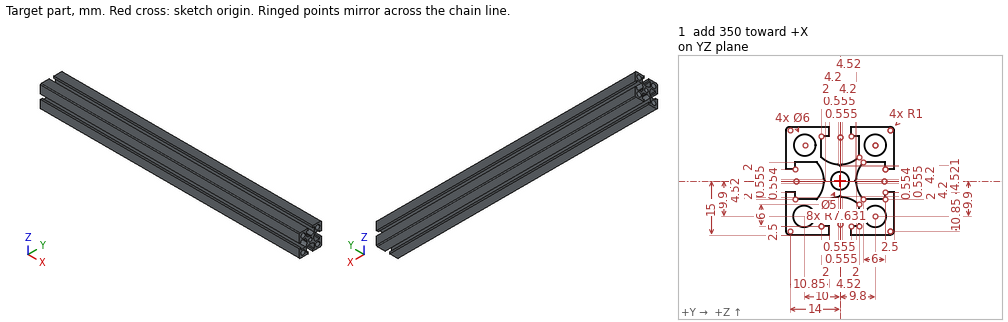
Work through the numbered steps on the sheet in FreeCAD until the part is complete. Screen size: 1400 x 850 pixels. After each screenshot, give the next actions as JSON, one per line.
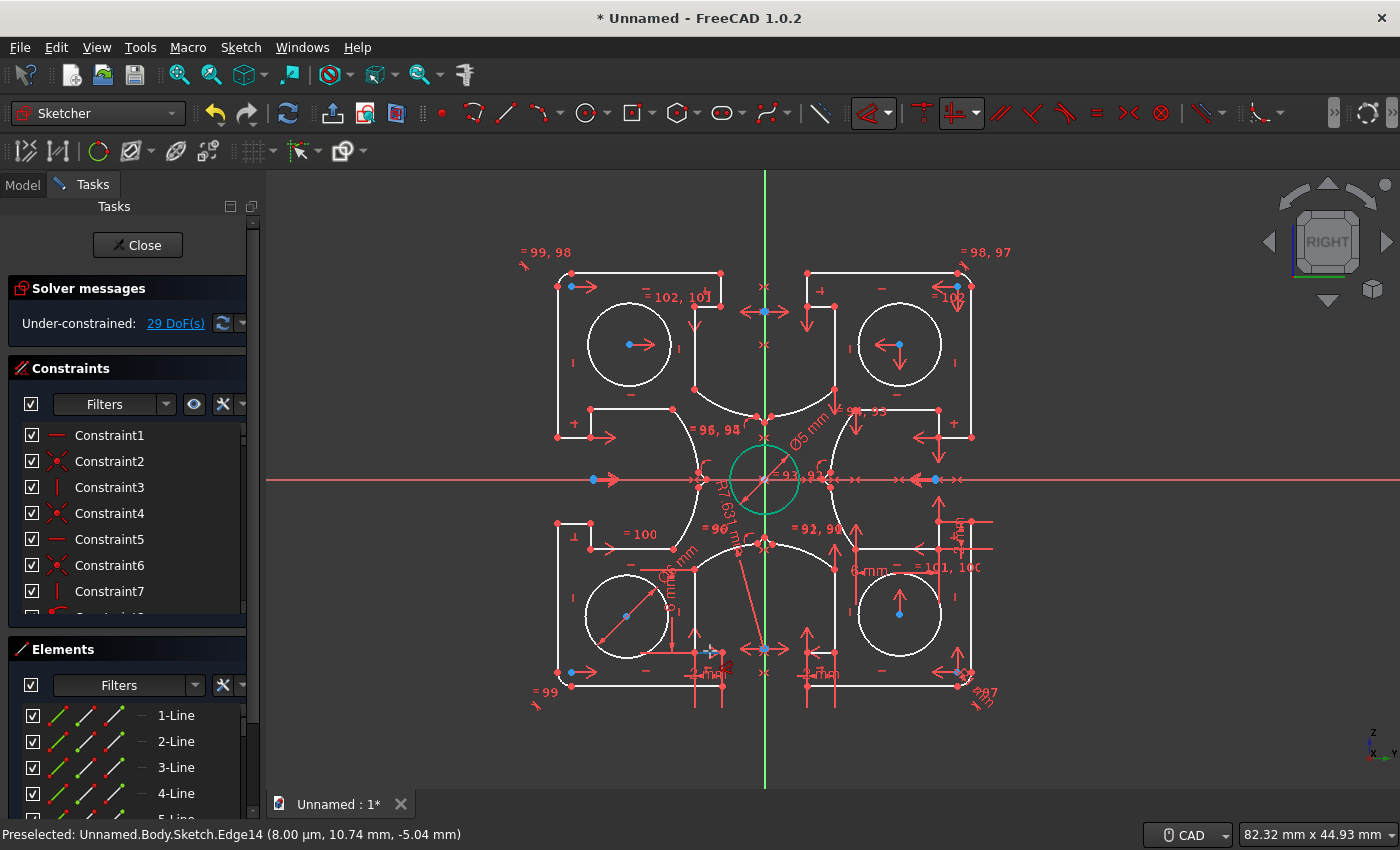
{"action": "scroll", "coordinate": [702, 307], "scroll_direction": "up", "scroll_amount": 3}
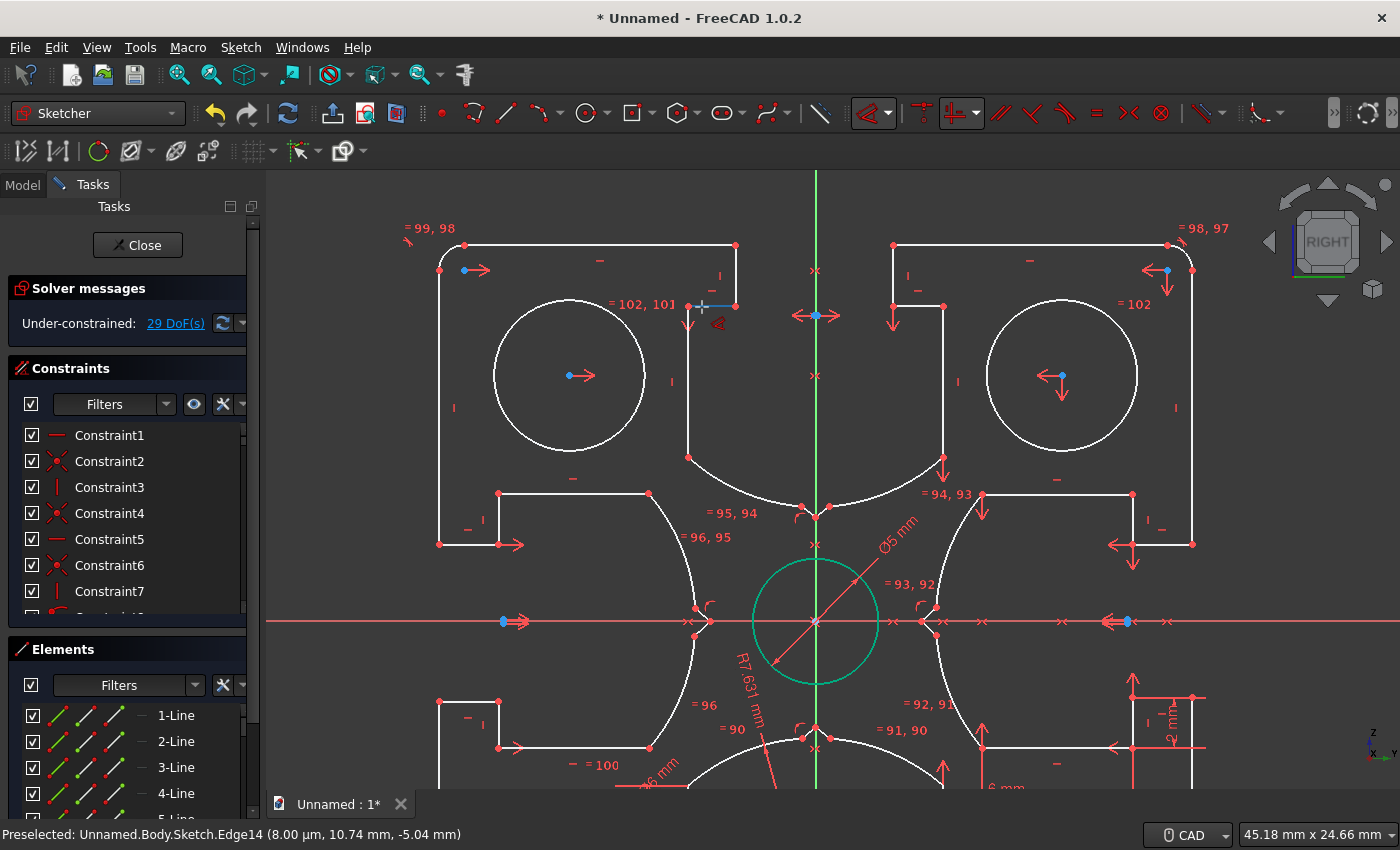
{"action": "left_click", "coordinate": [703, 306]}
{"action": "left_click", "coordinate": [712, 272]}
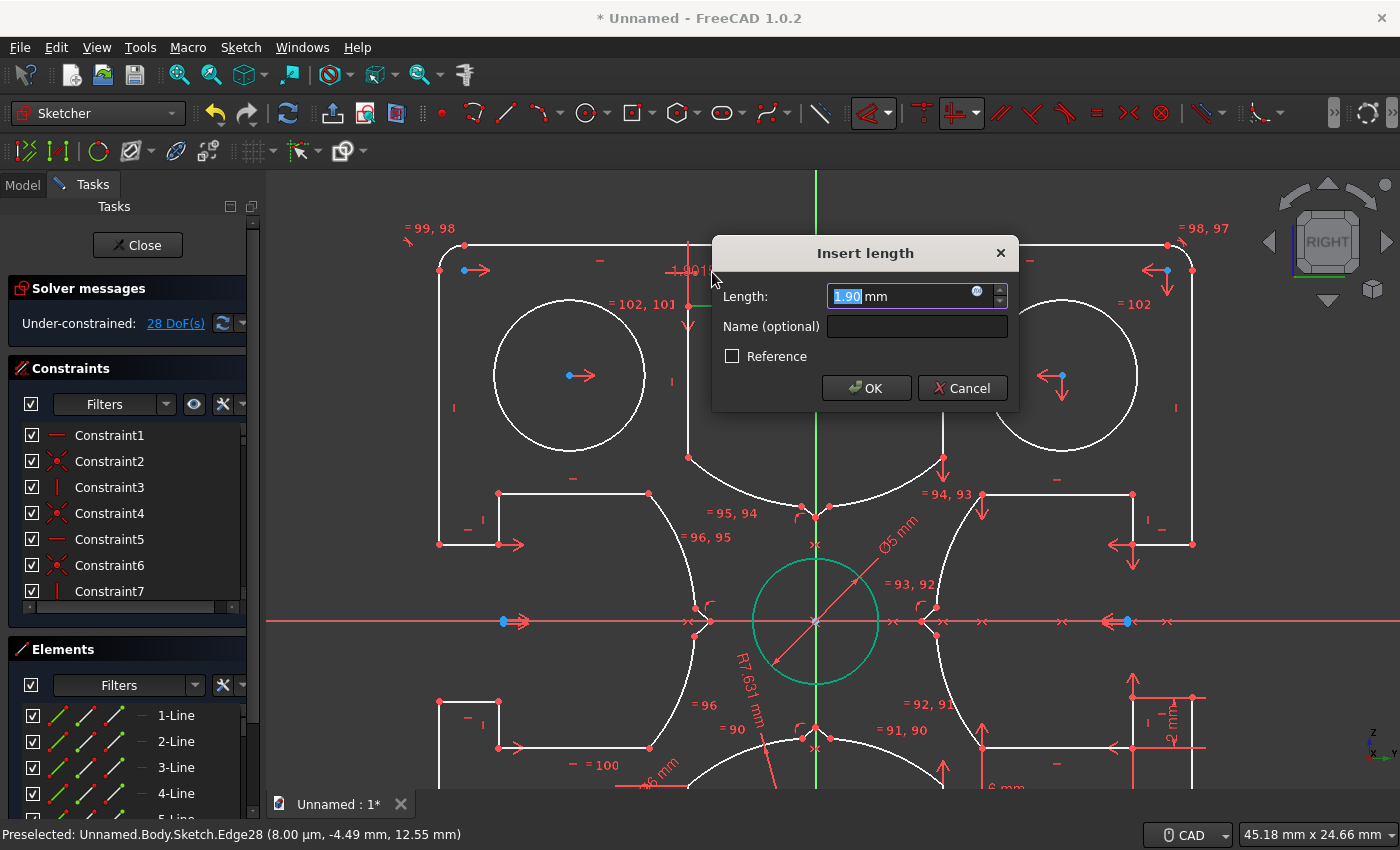
{"action": "type", "text": "2"}
{"action": "key", "text": "Return"}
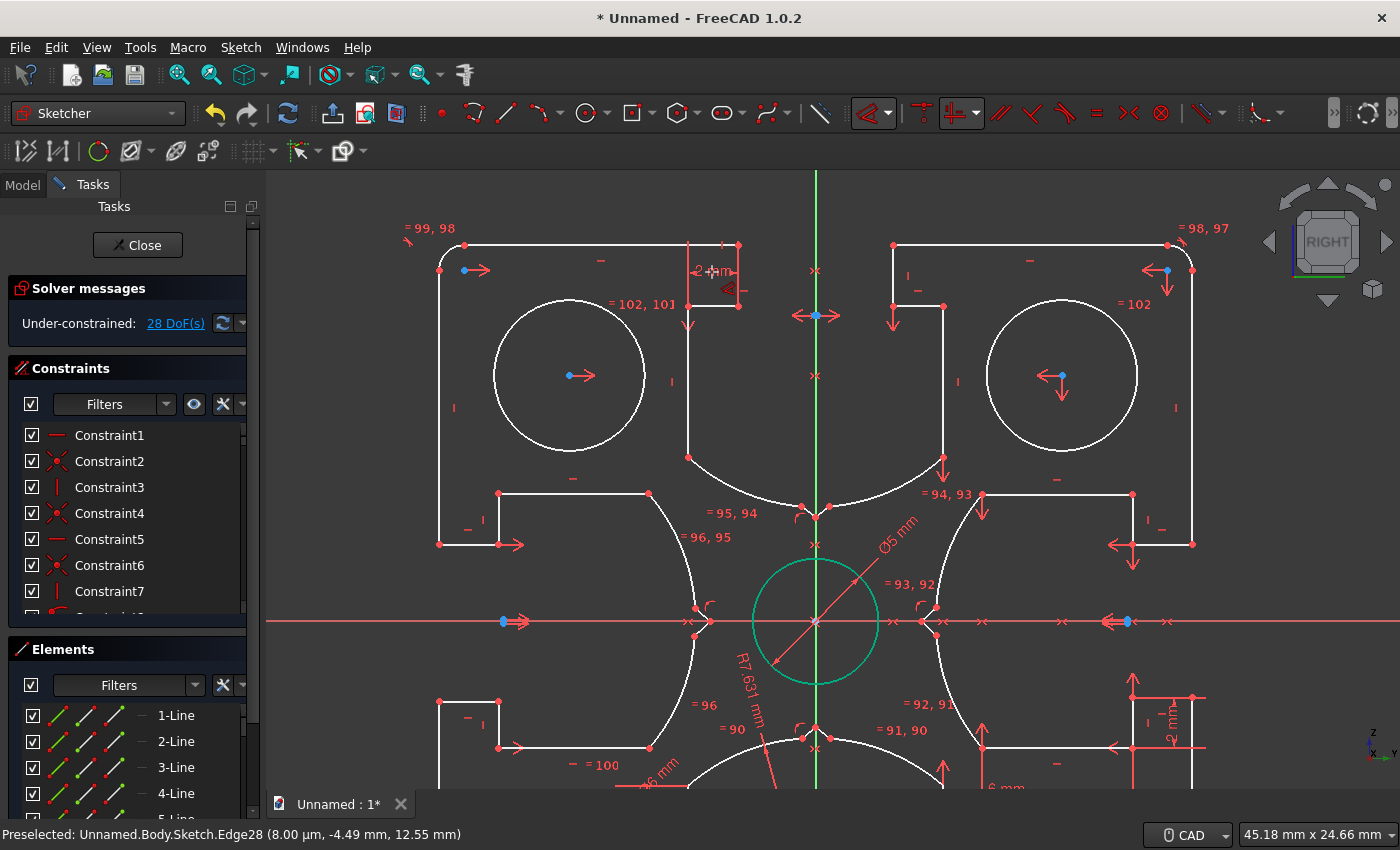
{"action": "left_click", "coordinate": [499, 530]}
{"action": "left_click", "coordinate": [465, 519]}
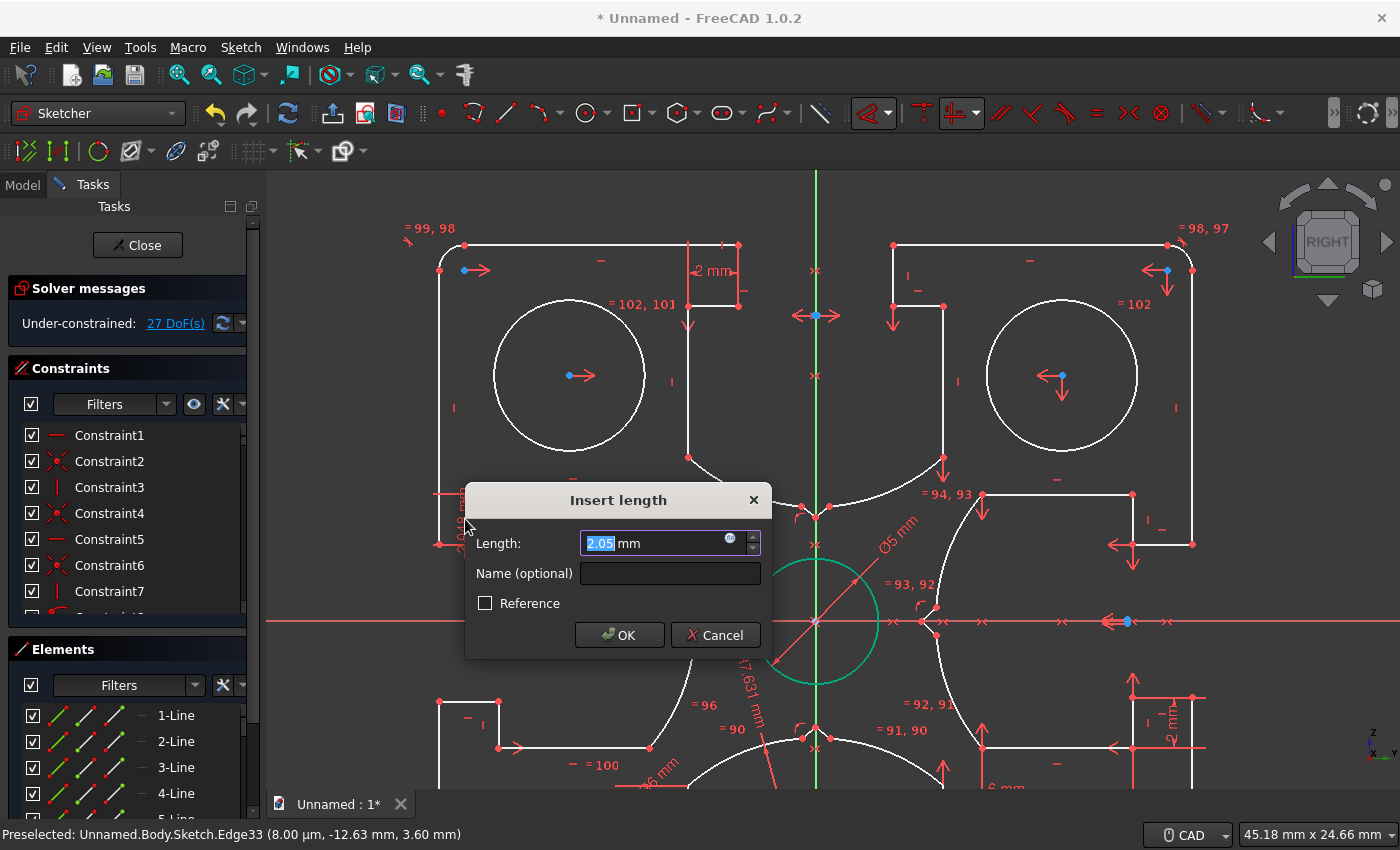
{"action": "type", "text": "2"}
{"action": "key", "text": "Return"}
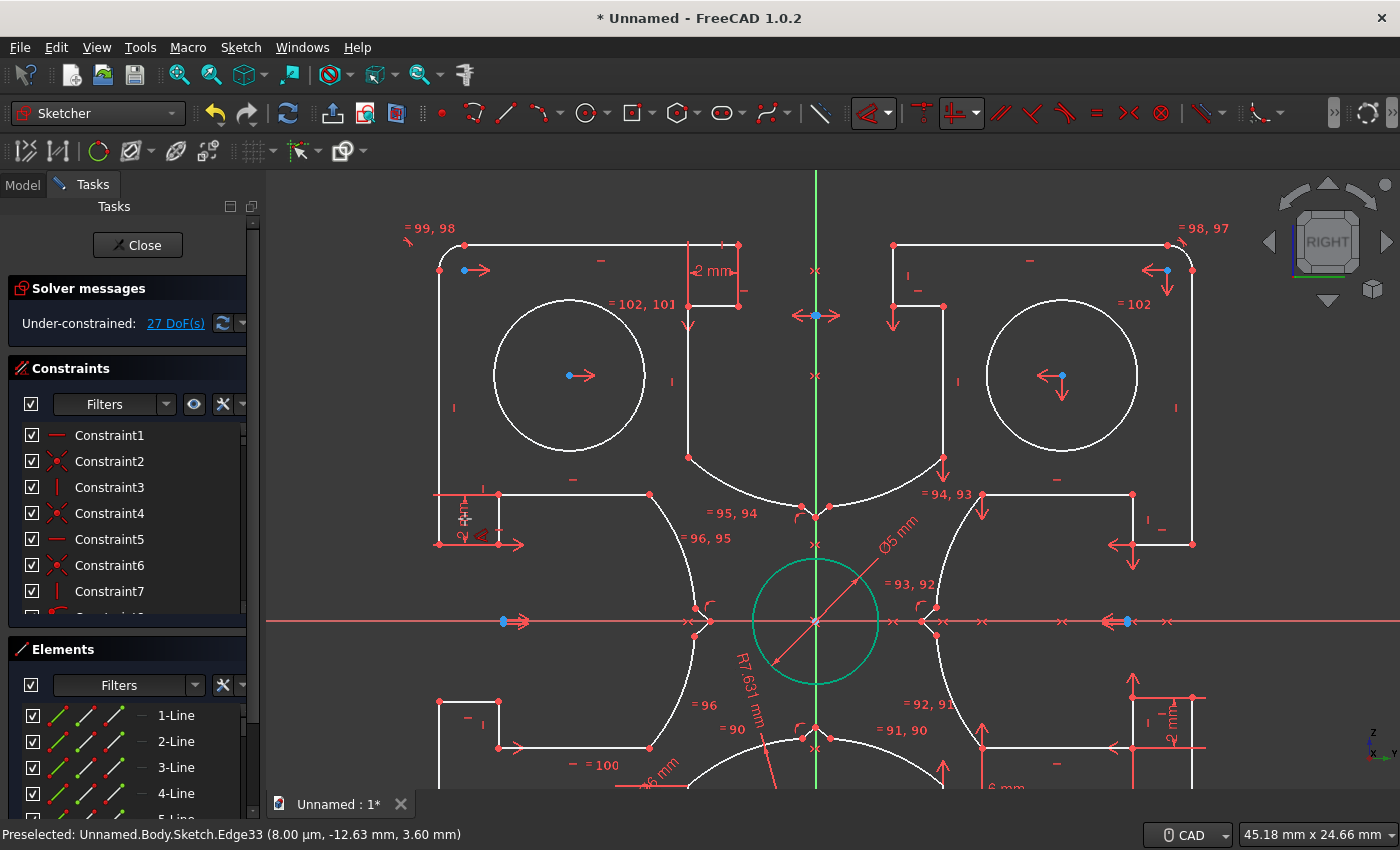
{"action": "left_click", "coordinate": [499, 734]}
{"action": "left_click", "coordinate": [465, 725]}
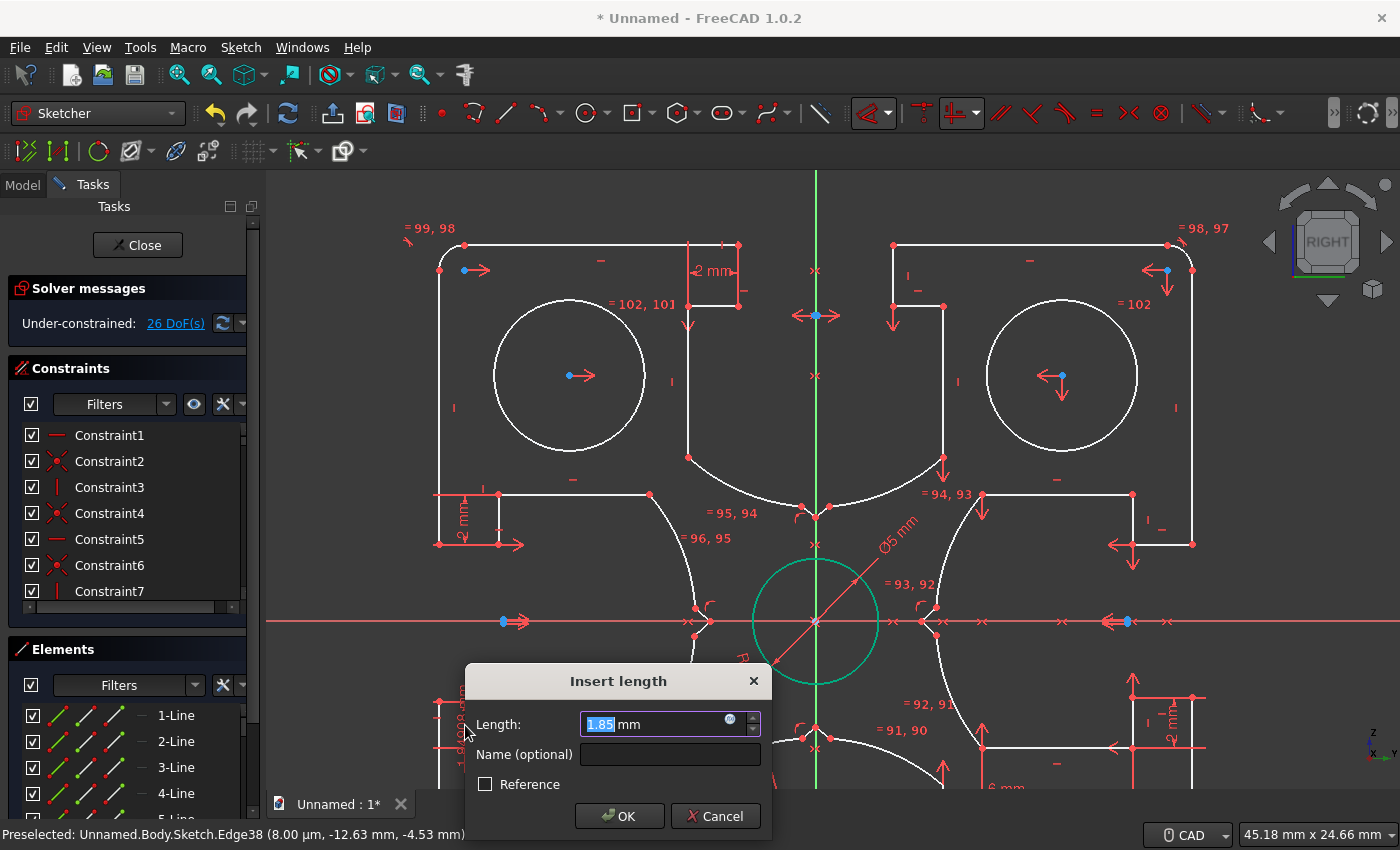
{"action": "type", "text": "2"}
{"action": "key", "text": "Return"}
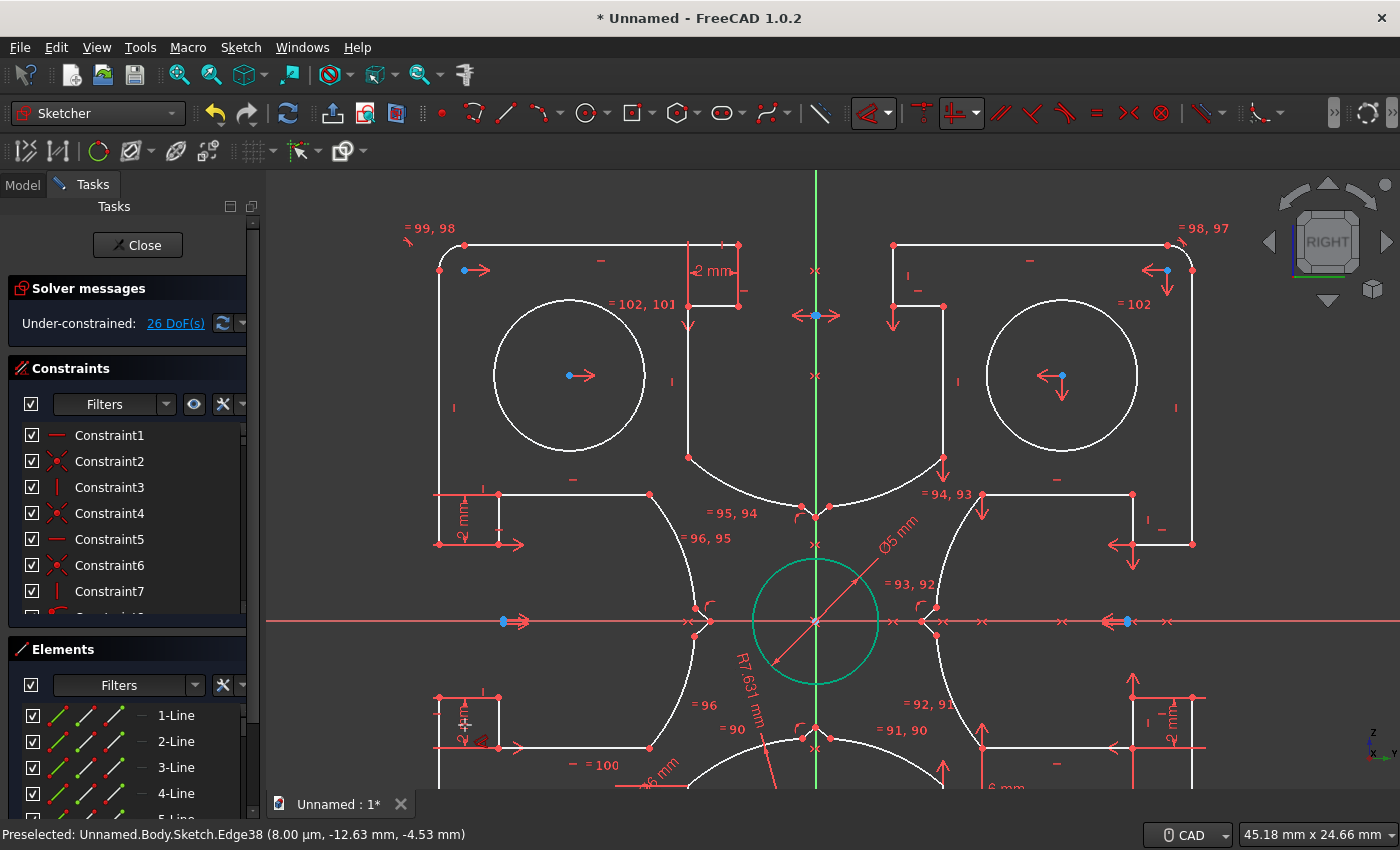
{"action": "scroll", "coordinate": [702, 307], "scroll_direction": "down", "scroll_amount": 3}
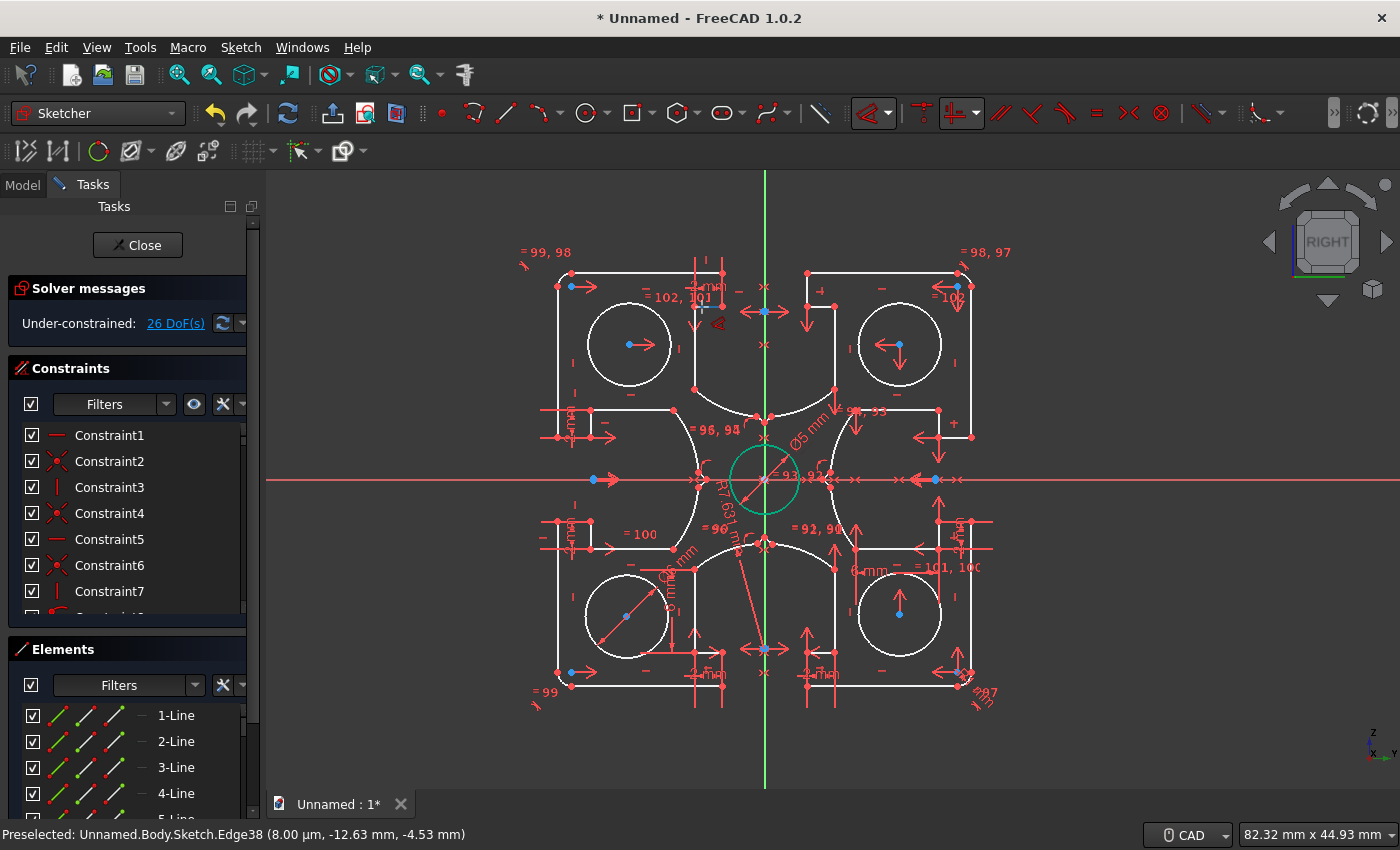
{"action": "left_click", "coordinate": [627, 617]}
{"action": "left_click", "coordinate": [744, 651]}